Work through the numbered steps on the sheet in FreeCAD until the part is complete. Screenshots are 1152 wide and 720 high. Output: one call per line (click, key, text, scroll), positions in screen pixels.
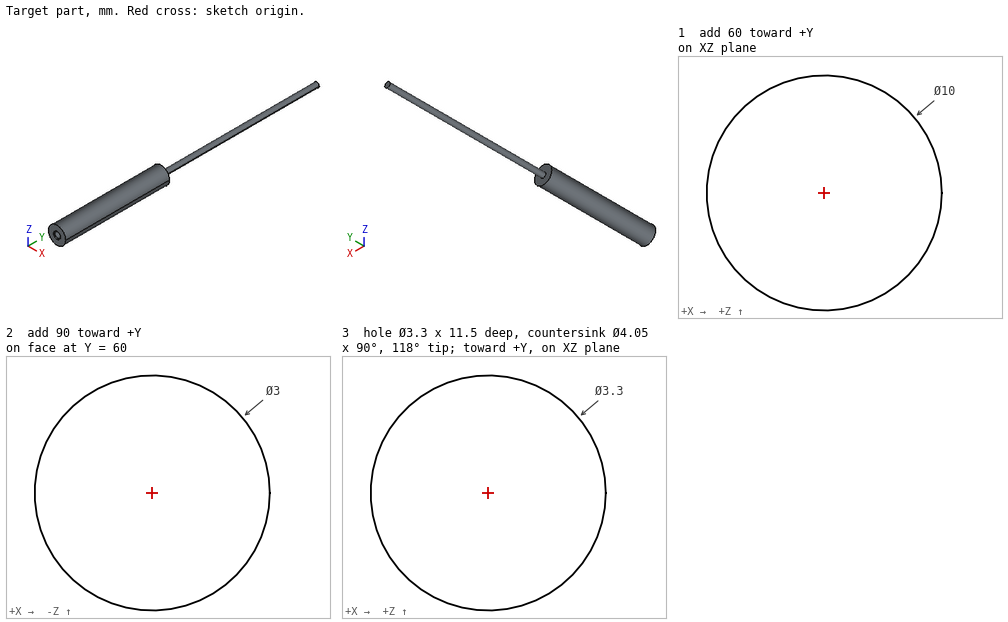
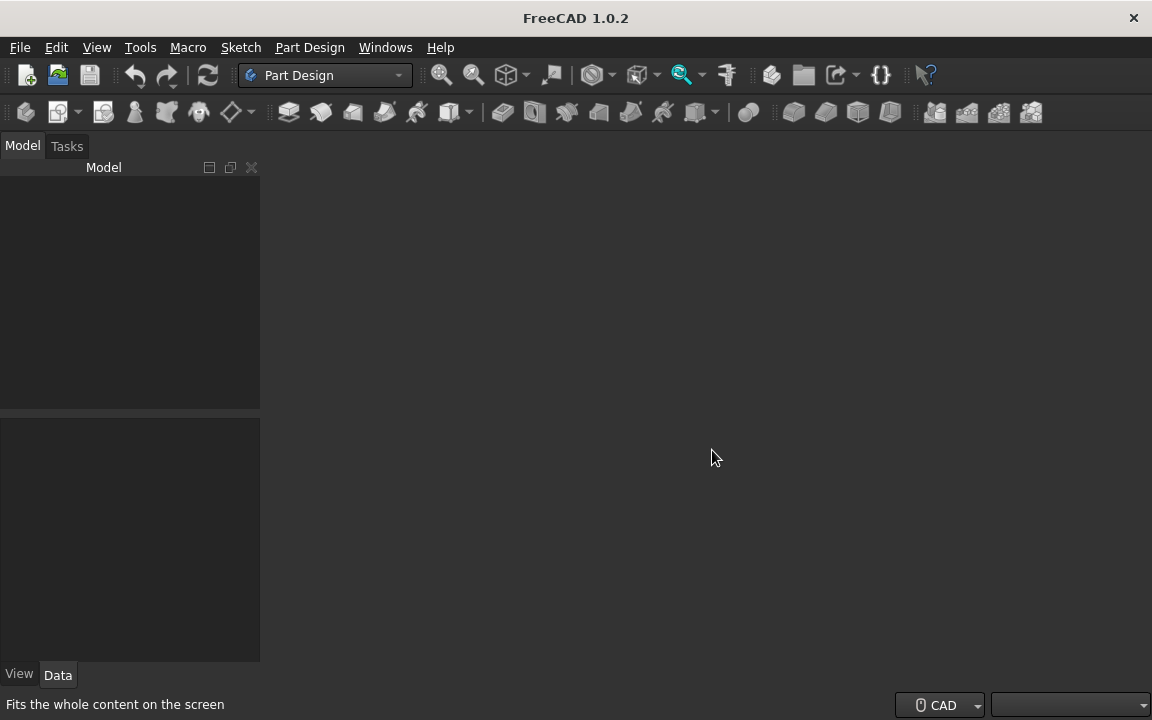
click(26, 76)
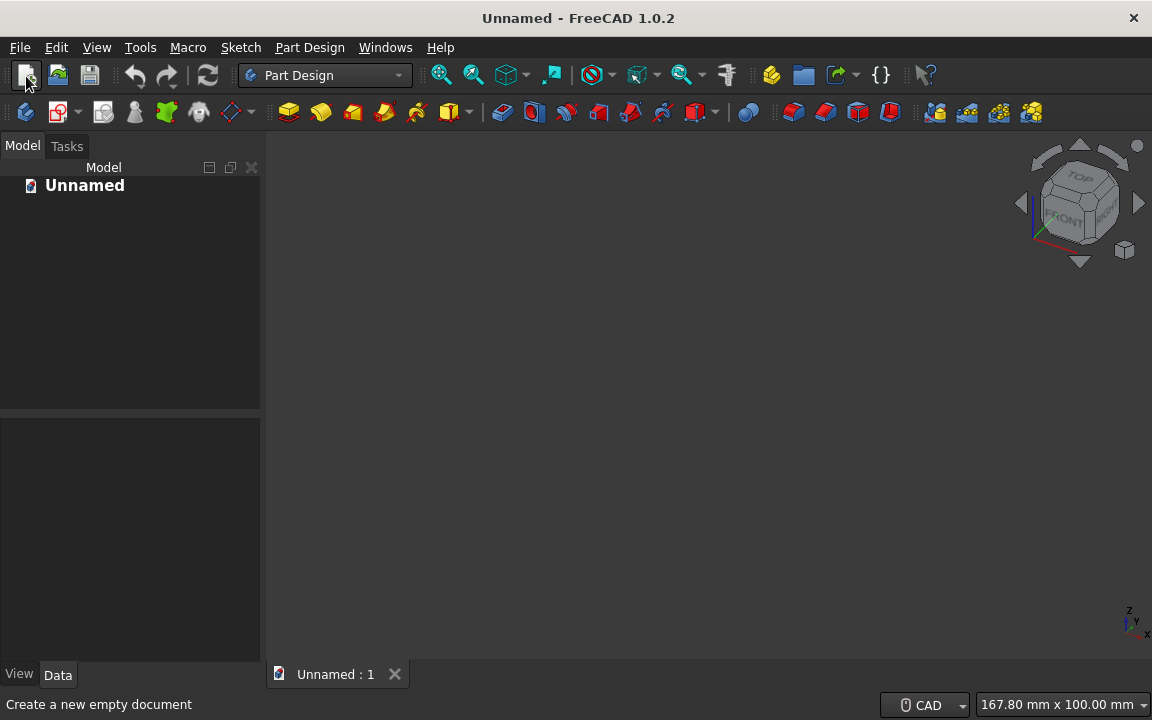
click(58, 112)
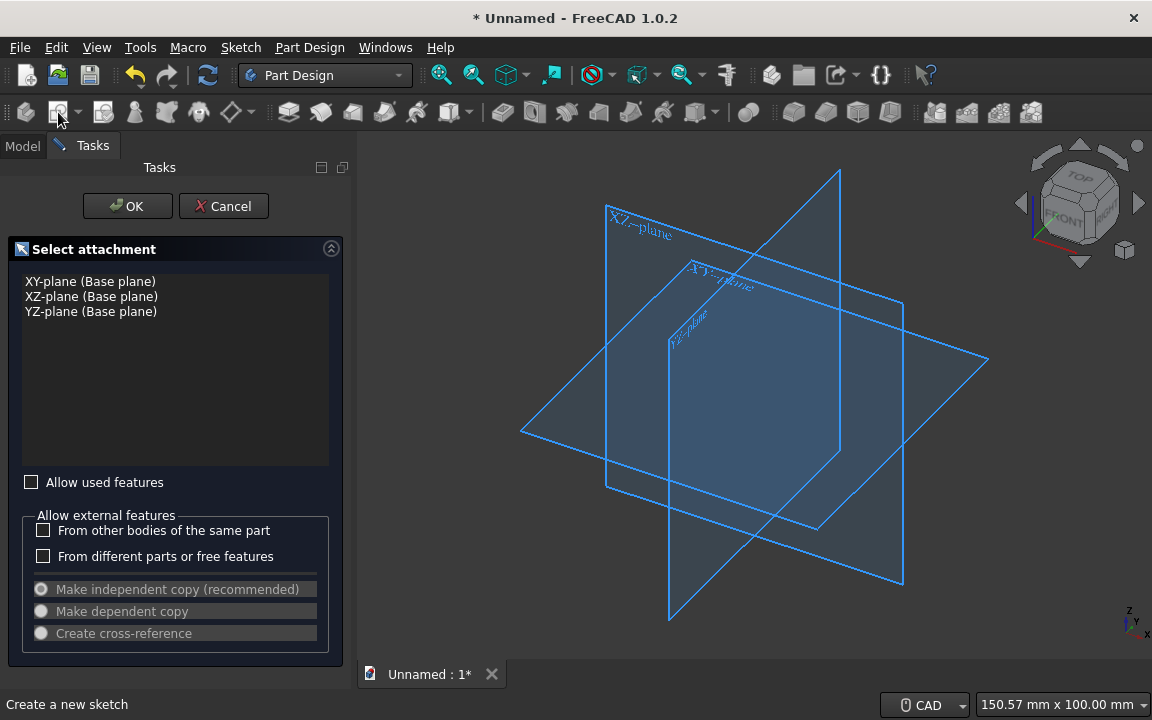
click(82, 296)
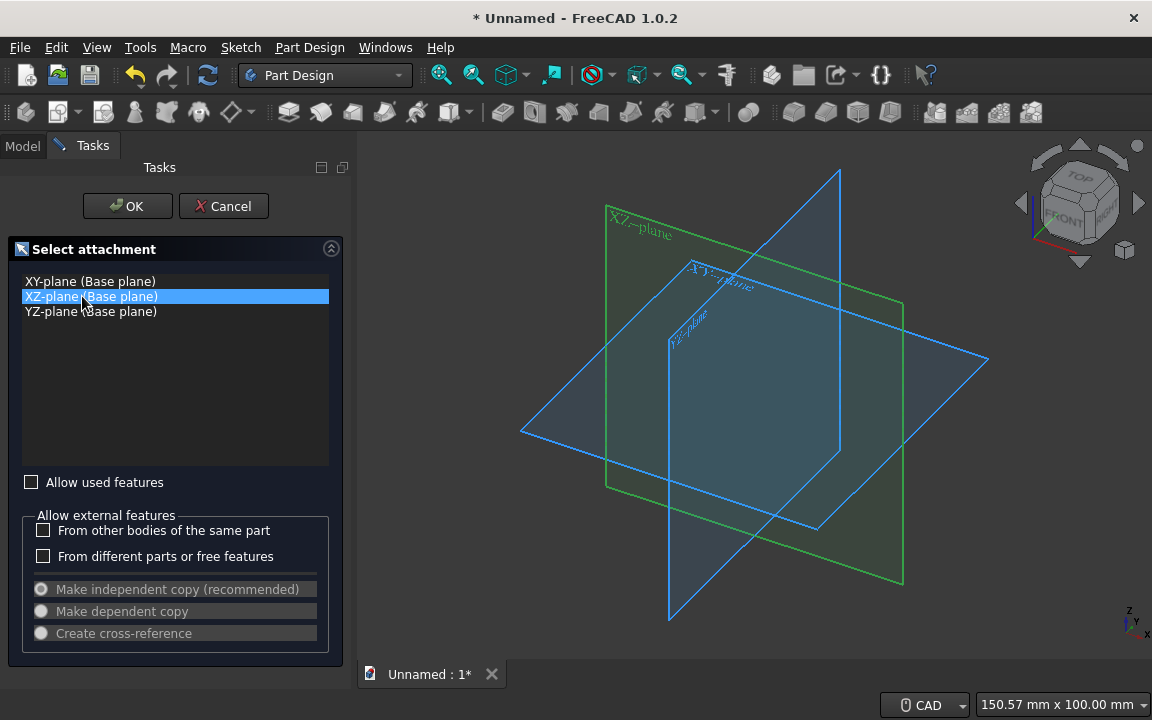
click(128, 206)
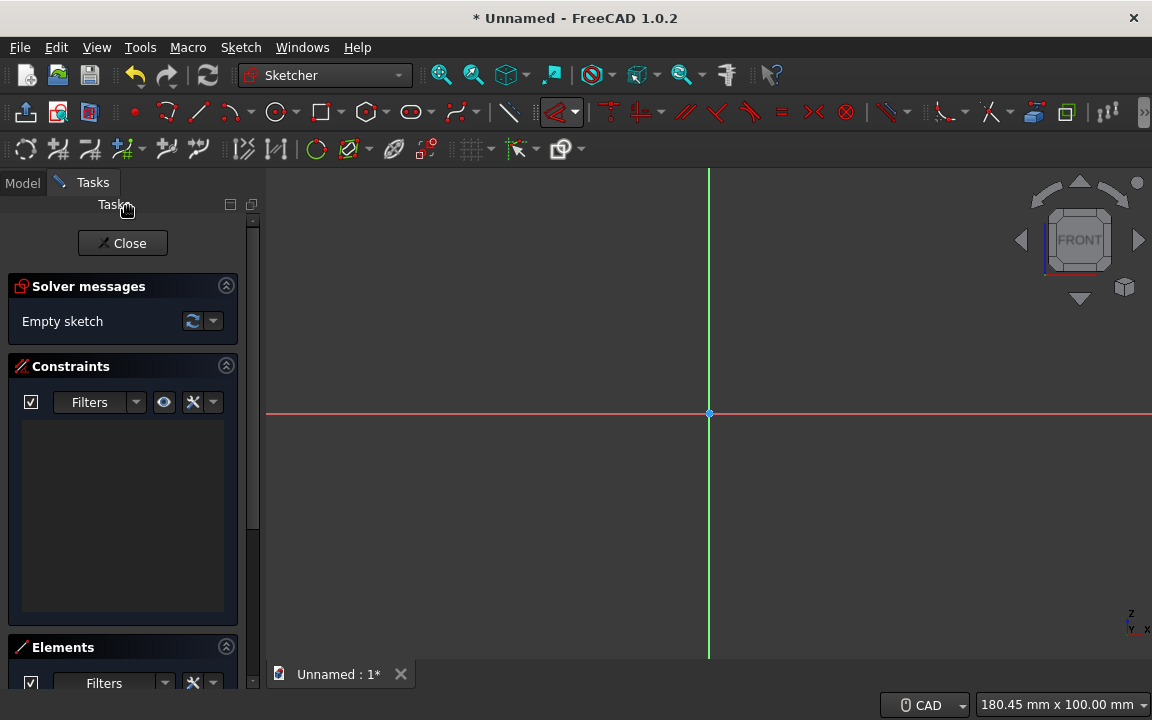
scroll(723, 414, up, 9)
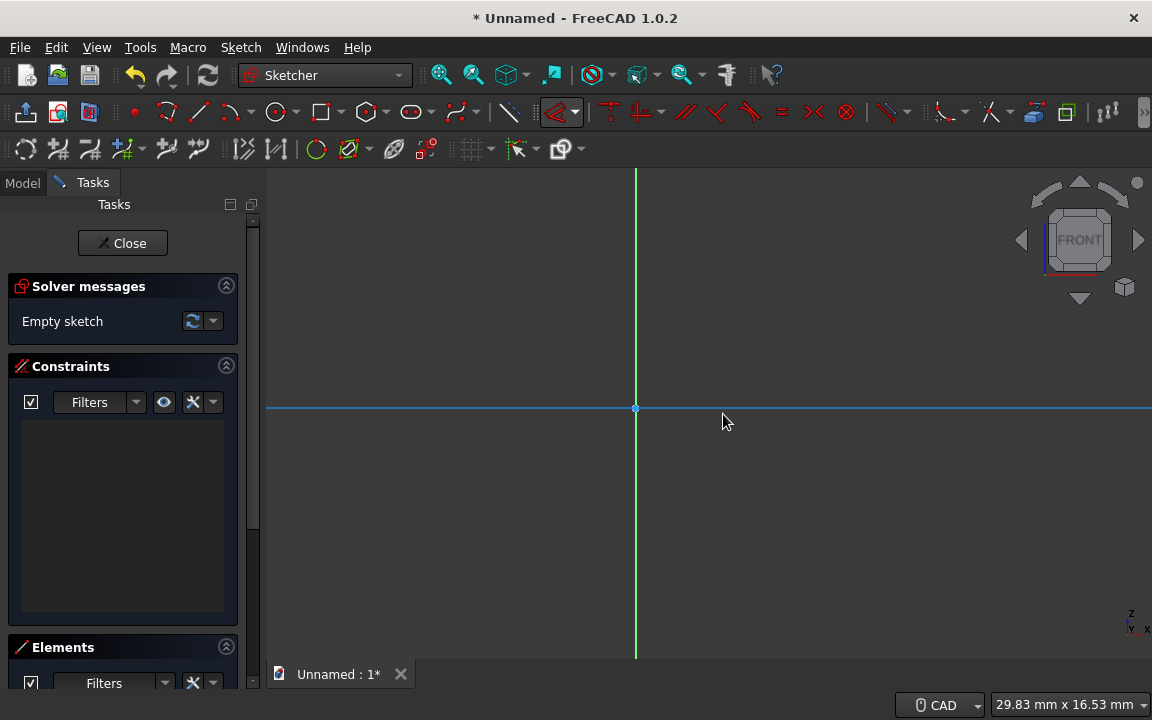
click(276, 112)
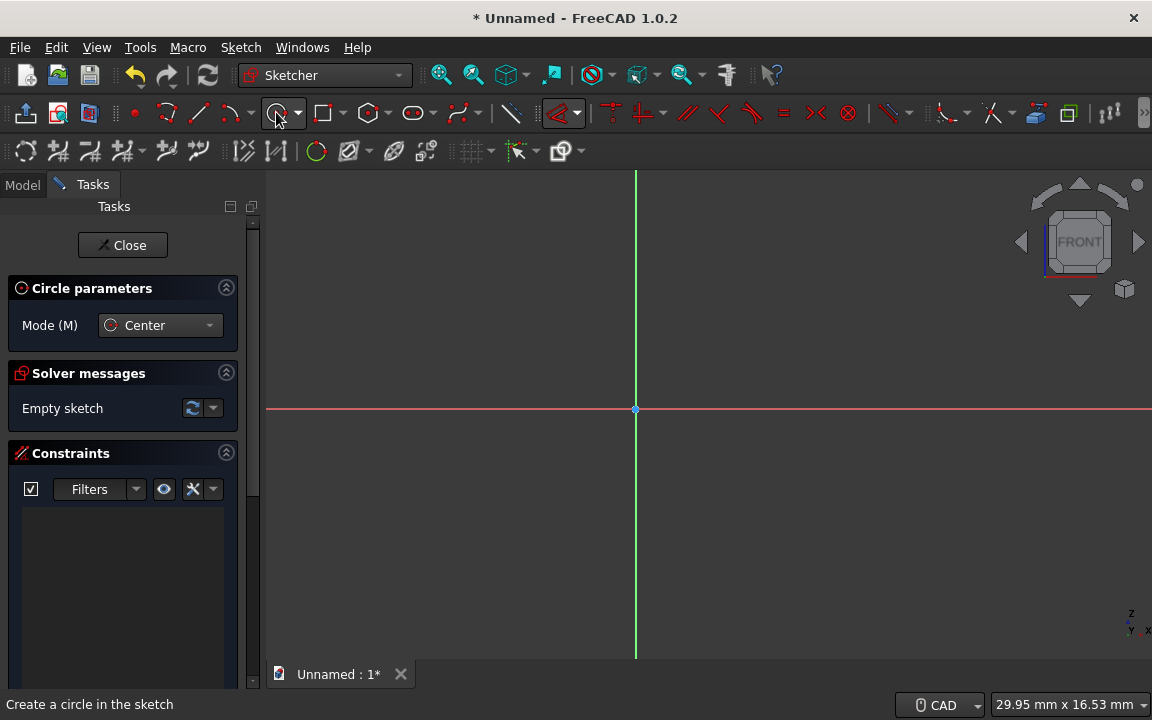
click(636, 409)
click(741, 305)
key(Escape)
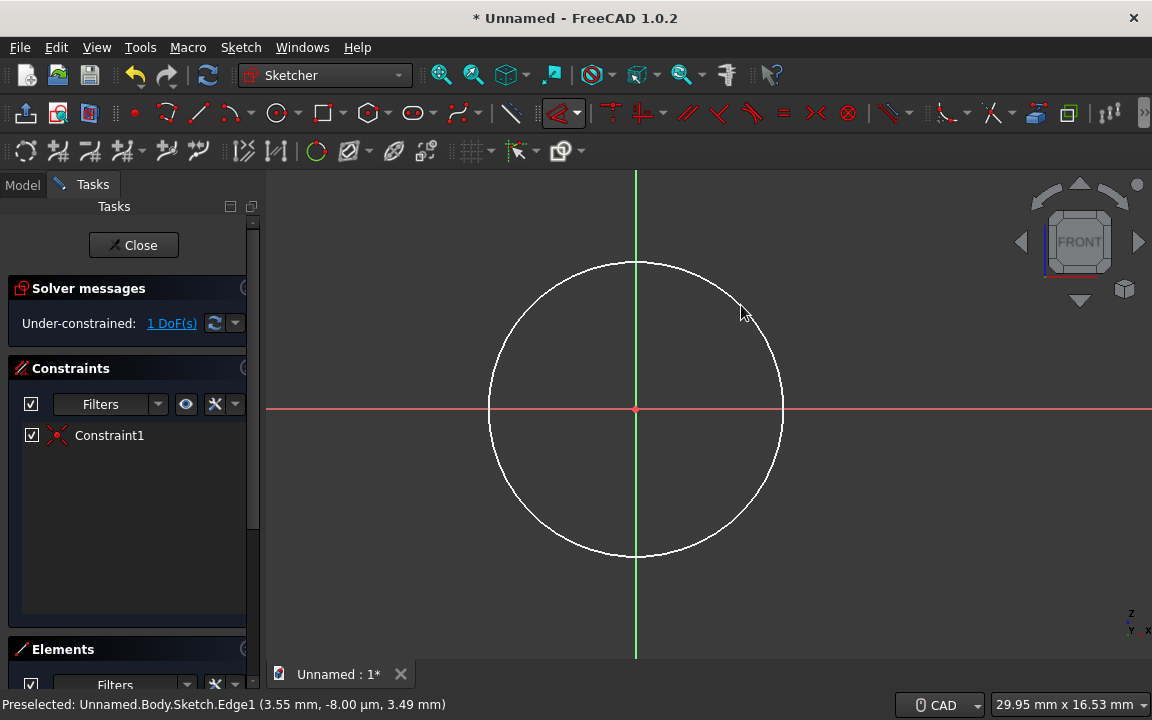
click(740, 305)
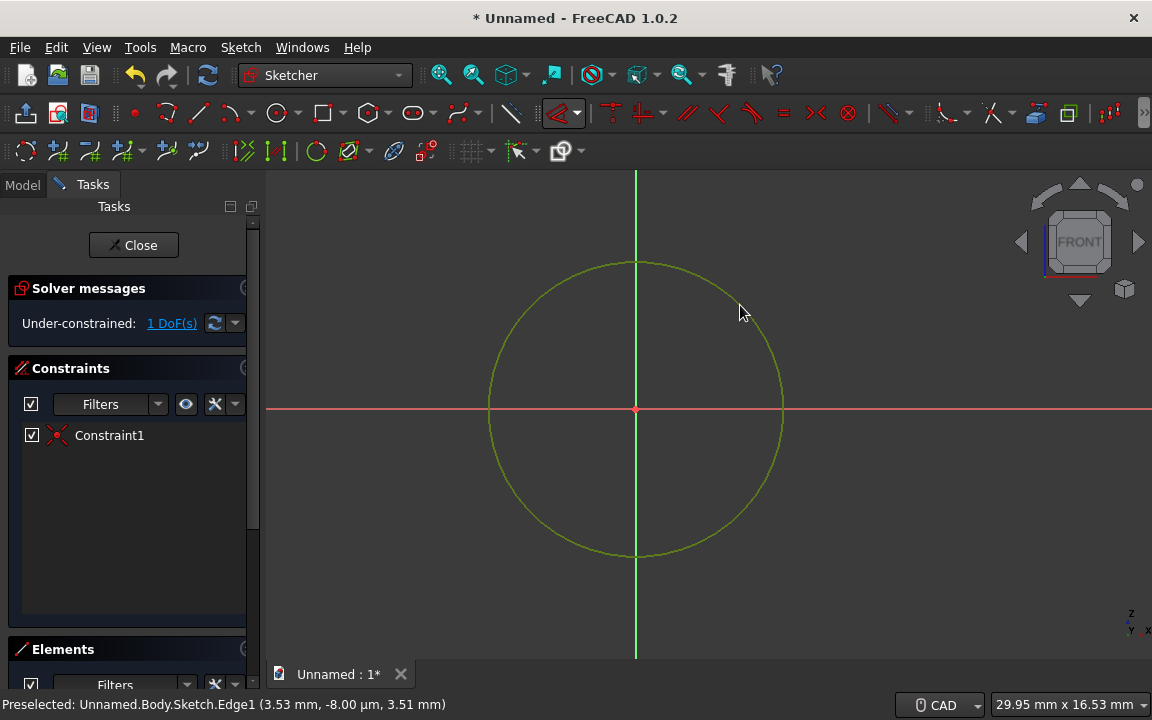
click(580, 114)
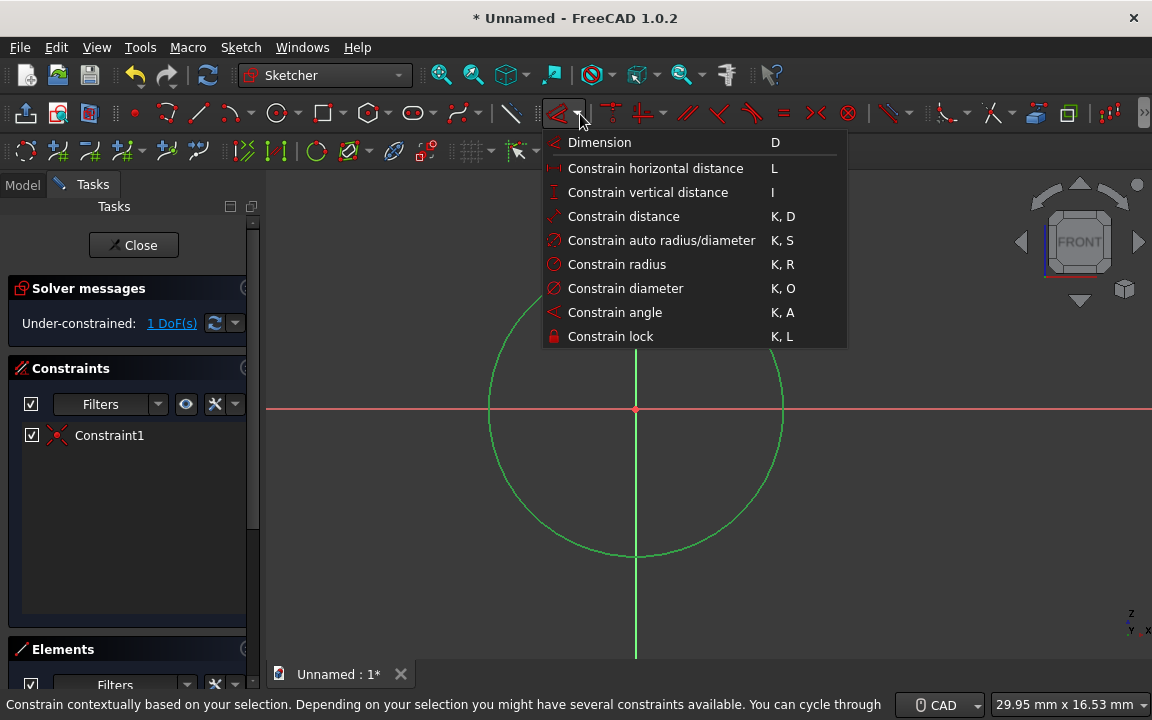
click(695, 288)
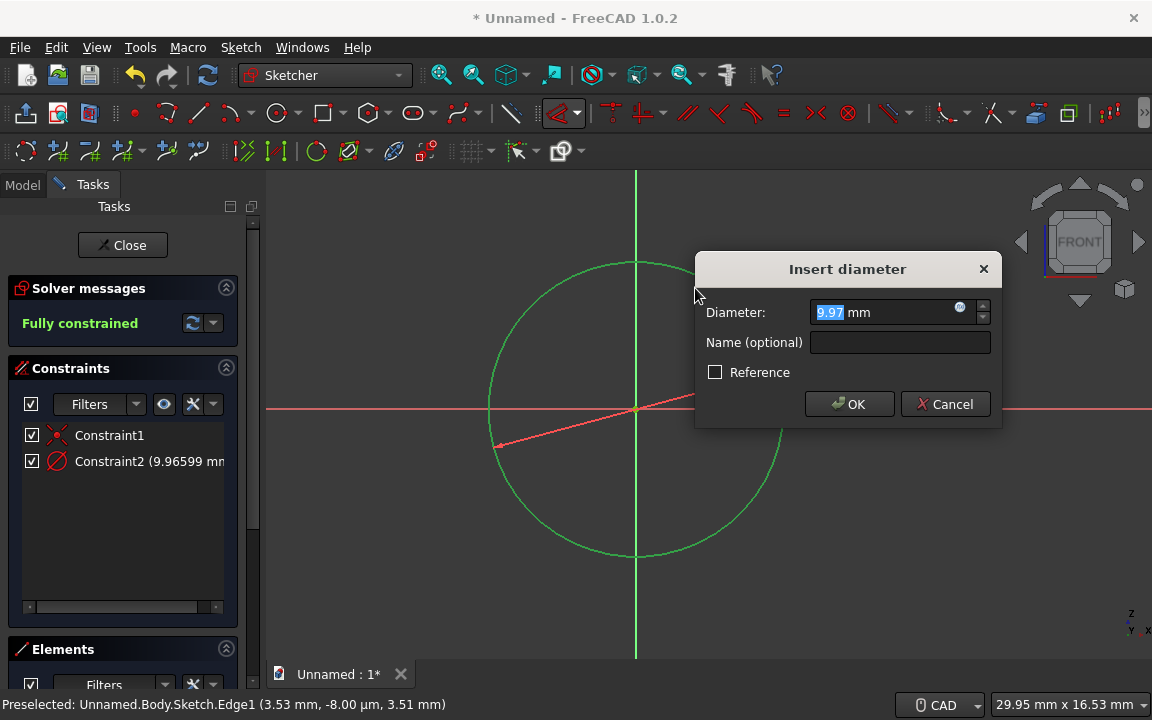
text(10)
key(Return)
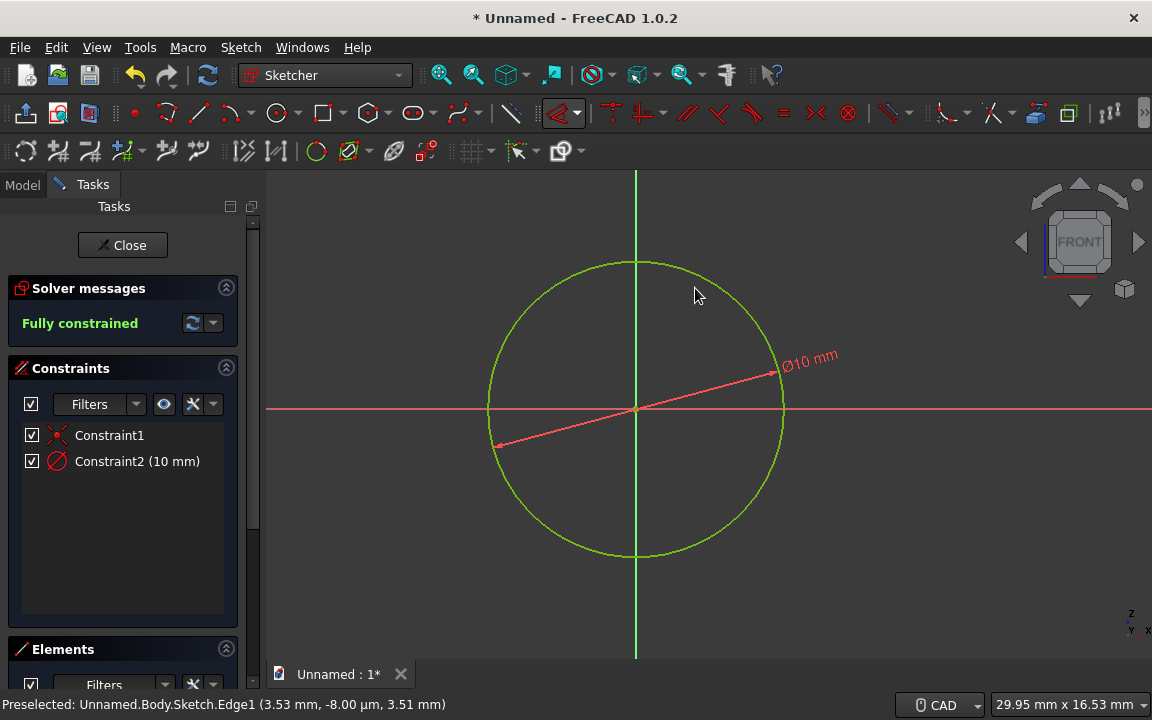
click(123, 245)